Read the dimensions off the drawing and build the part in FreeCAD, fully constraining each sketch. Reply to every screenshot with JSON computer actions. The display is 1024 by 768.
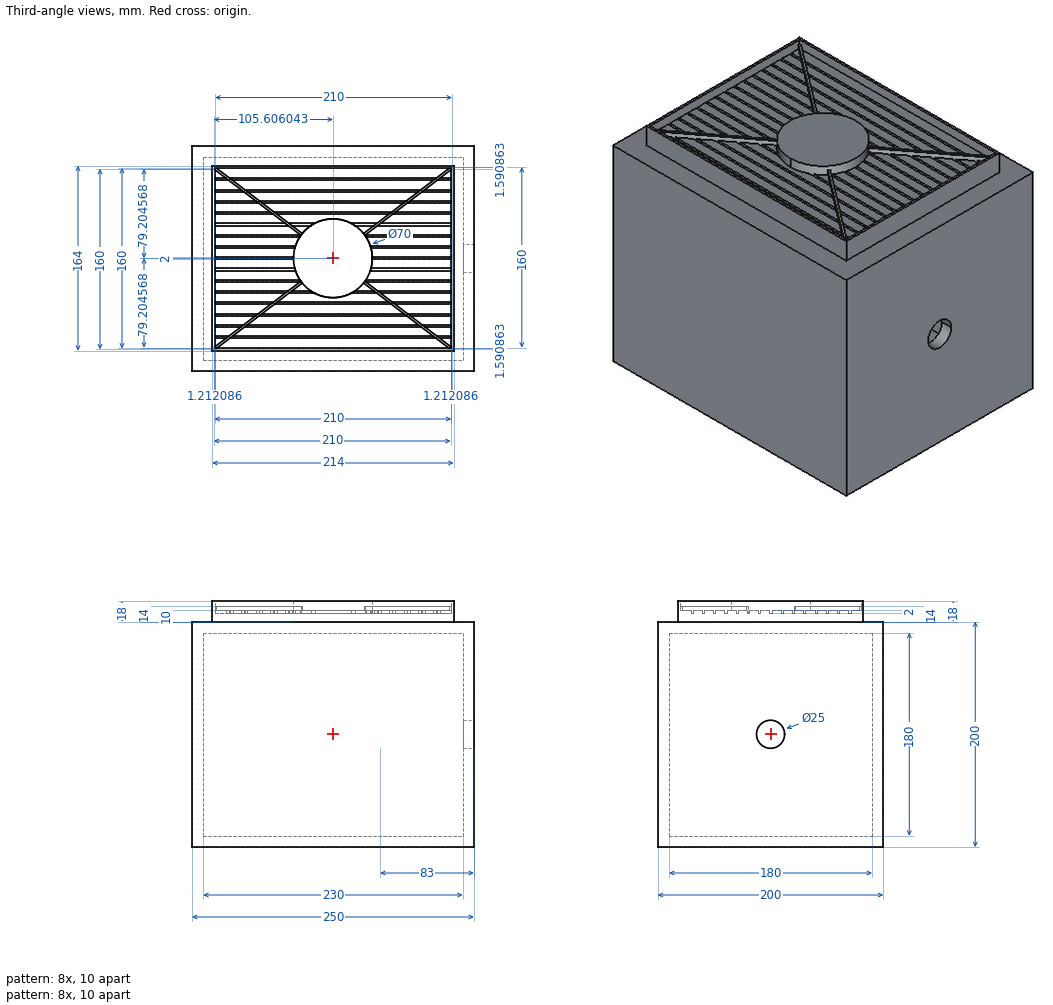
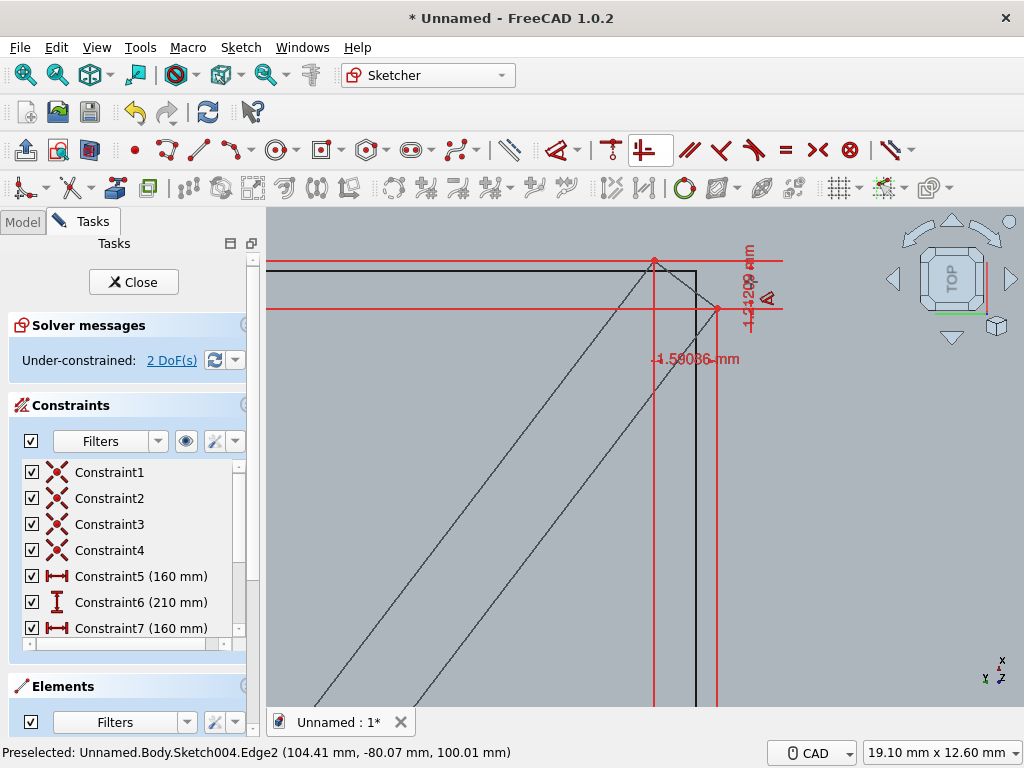
{"action": "scroll", "coordinate": [706, 288], "scroll_direction": "down", "scroll_amount": 16}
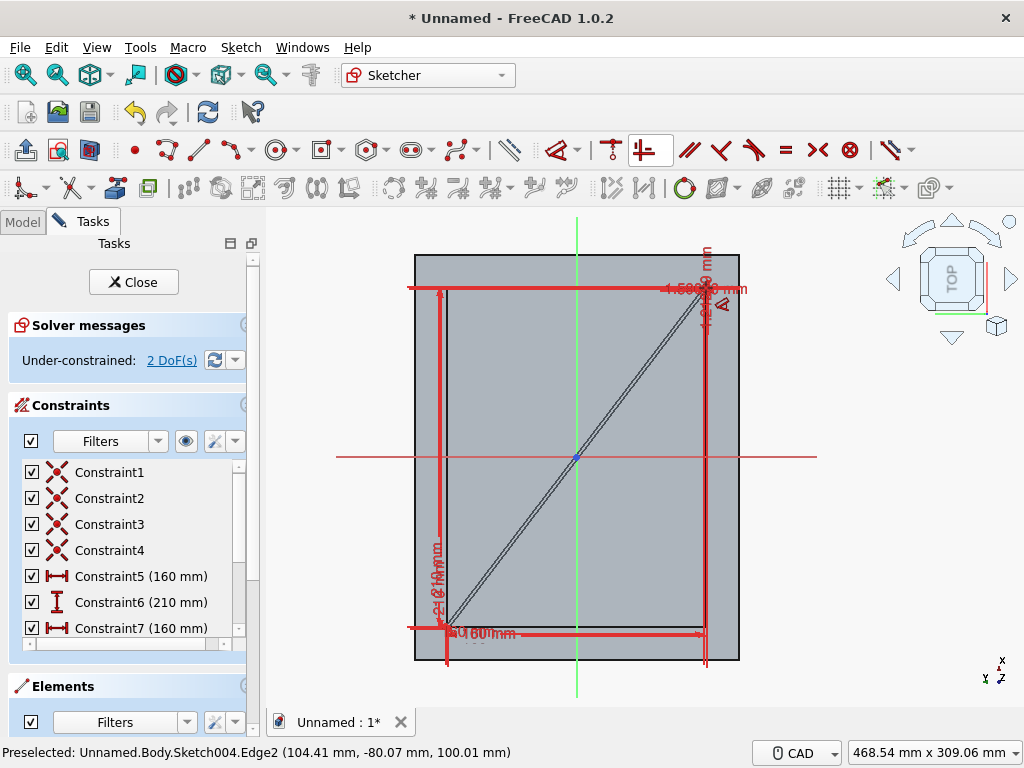
{"action": "scroll", "coordinate": [448, 629], "scroll_direction": "up", "scroll_amount": 7}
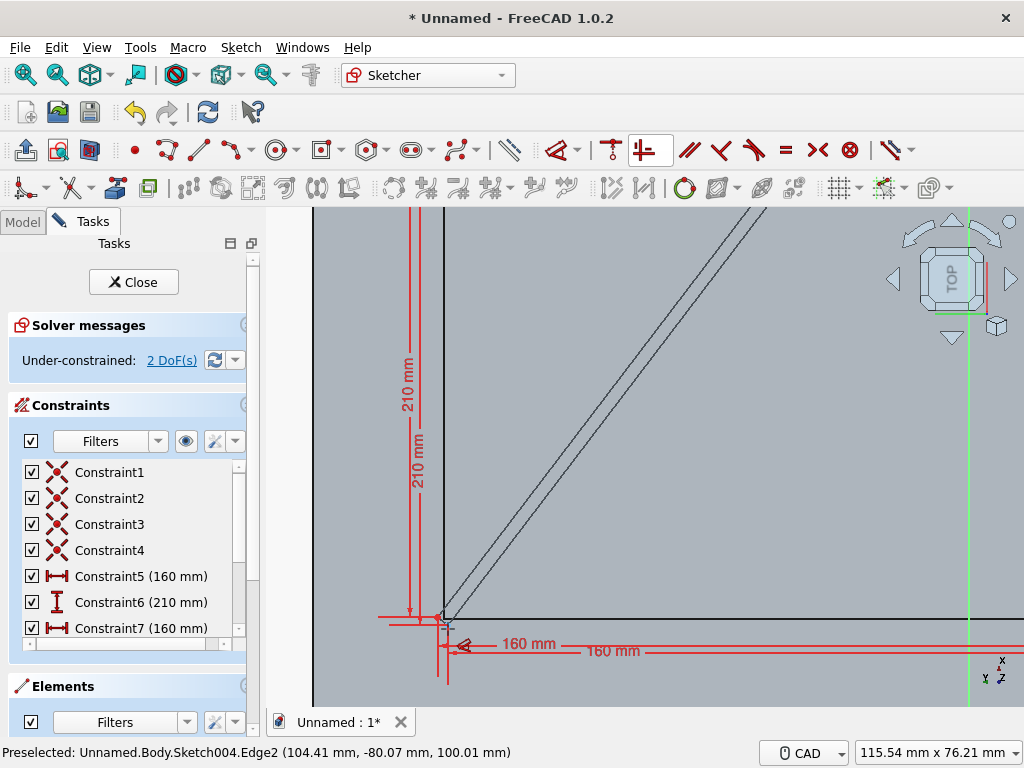
{"action": "left_click", "coordinate": [448, 625]}
{"action": "left_click", "coordinate": [748, 659]}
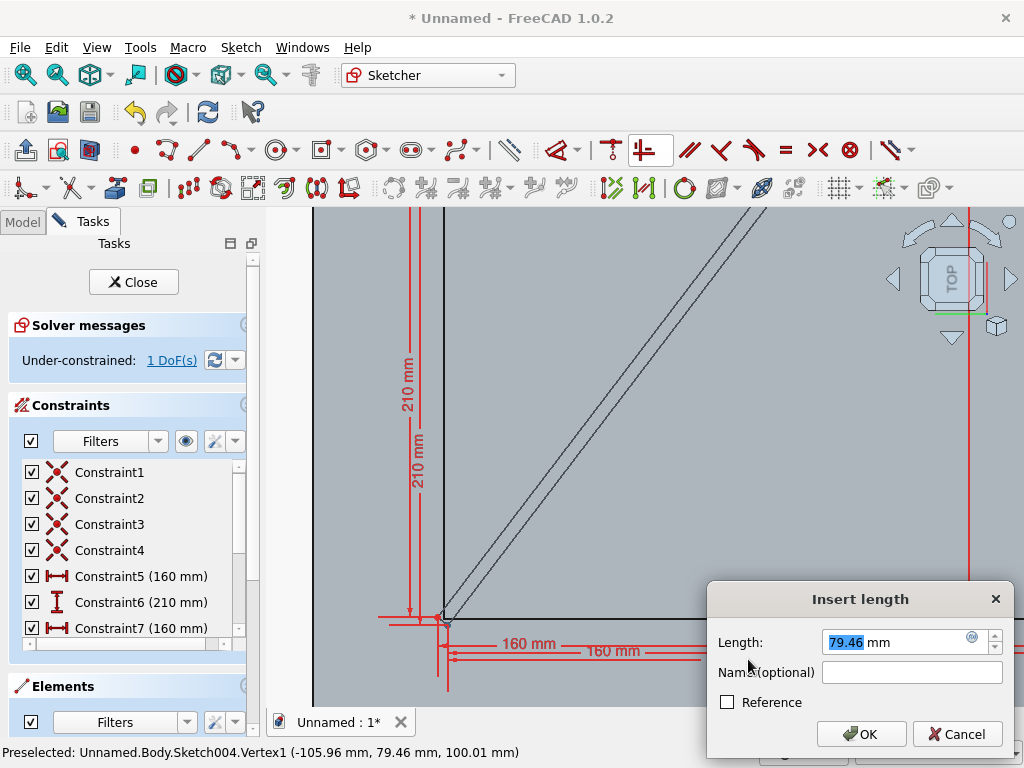
{"action": "type", "text": "79.204568"}
{"action": "key", "text": "Return"}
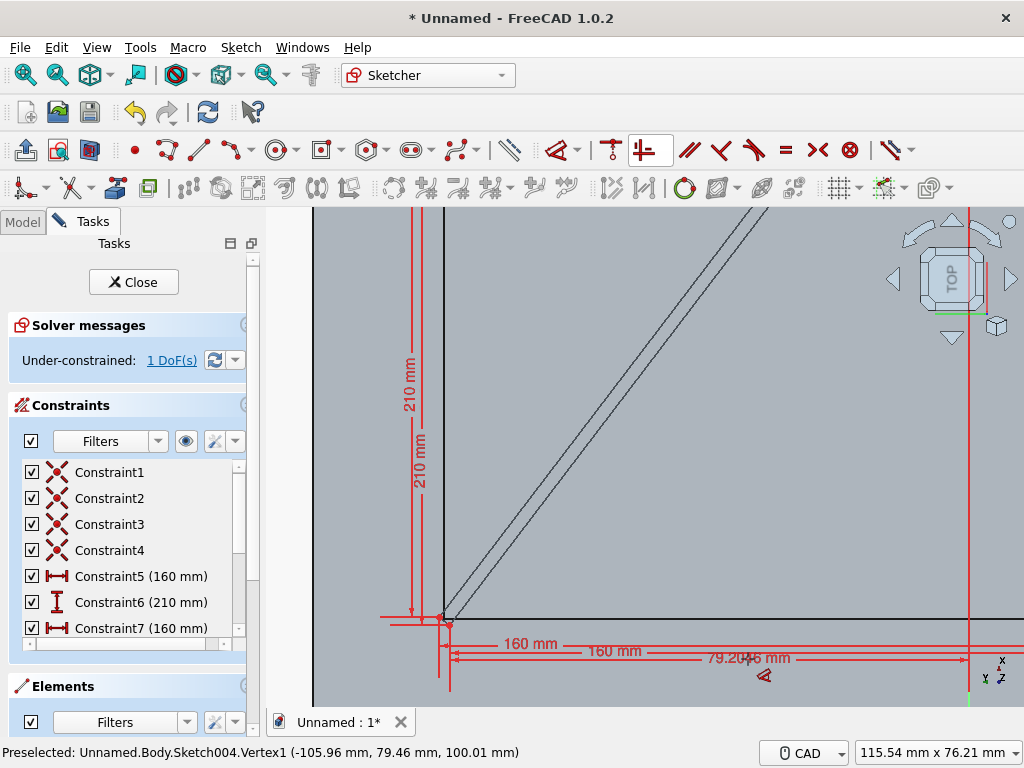
{"action": "left_click", "coordinate": [450, 625]}
{"action": "left_click", "coordinate": [416, 430]}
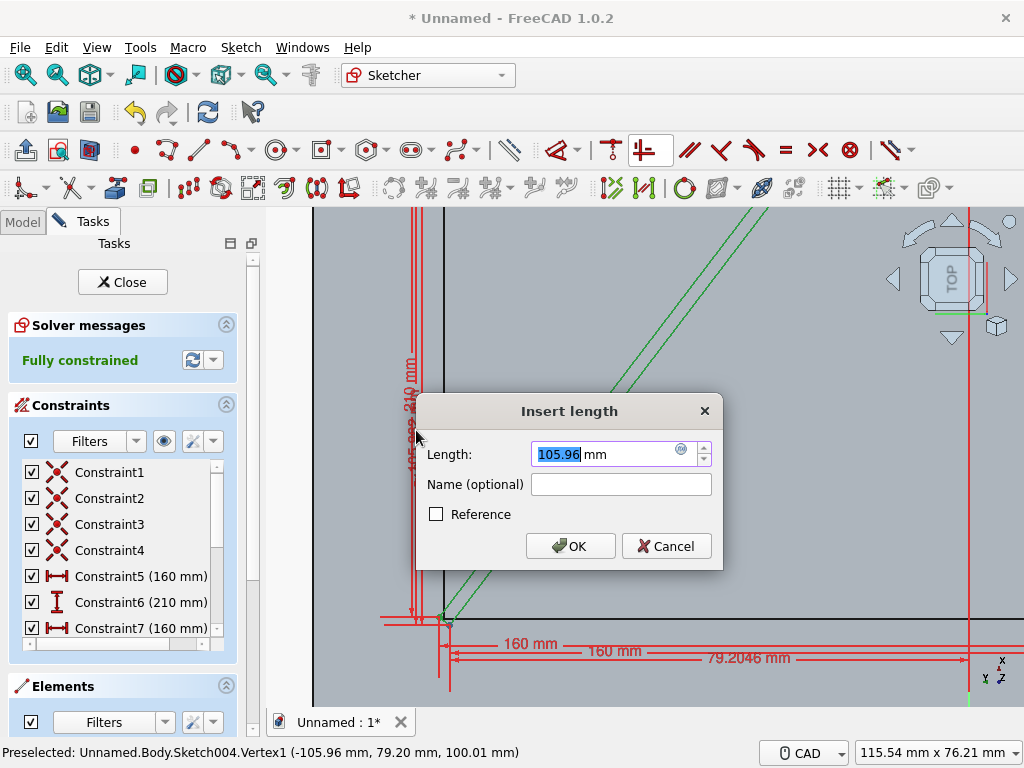
{"action": "type", "text": "105.606043"}
{"action": "key", "text": "Return"}
{"action": "key", "text": "Escape"}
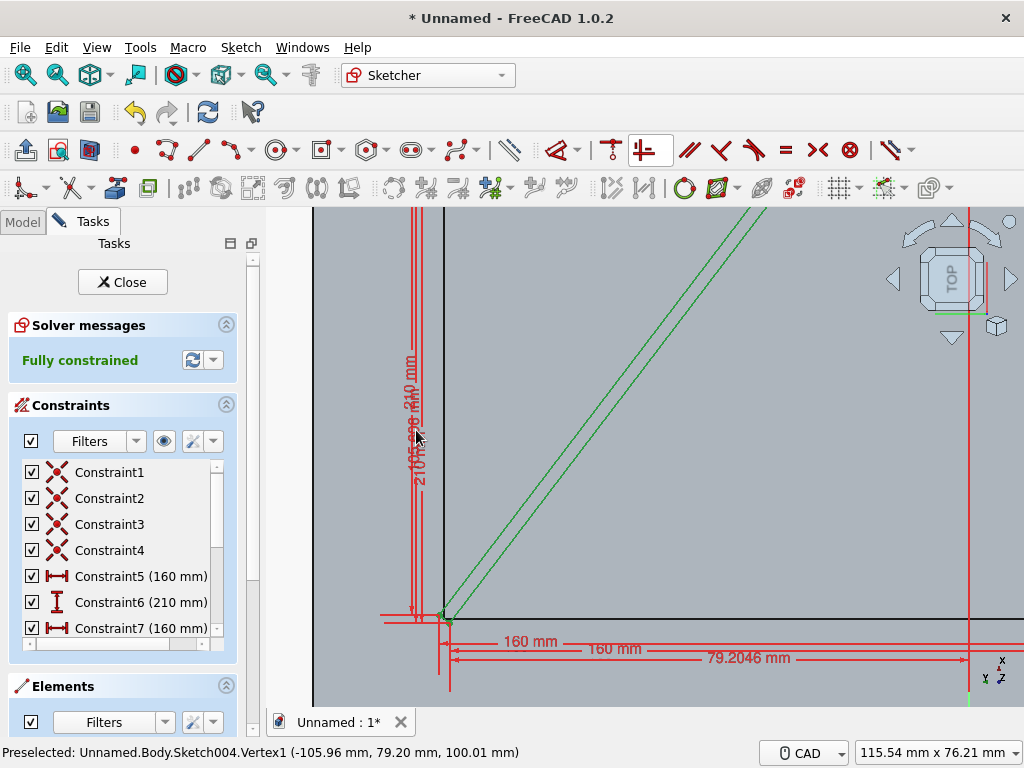
{"action": "left_click", "coordinate": [123, 282]}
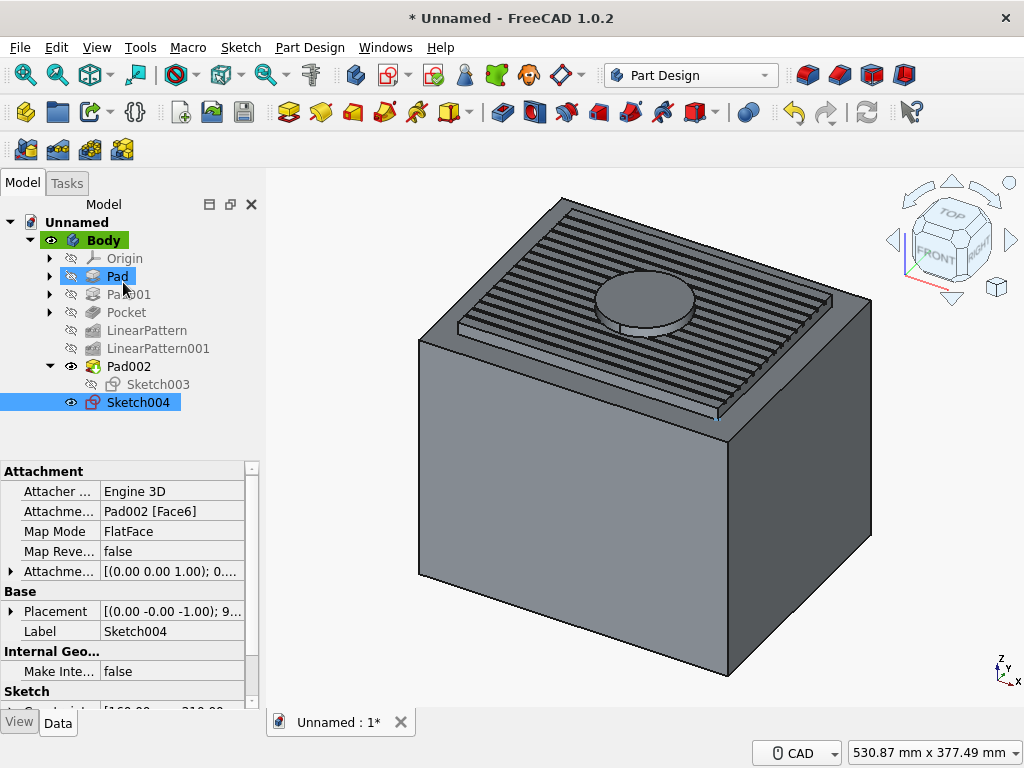
{"action": "left_click", "coordinate": [290, 112]}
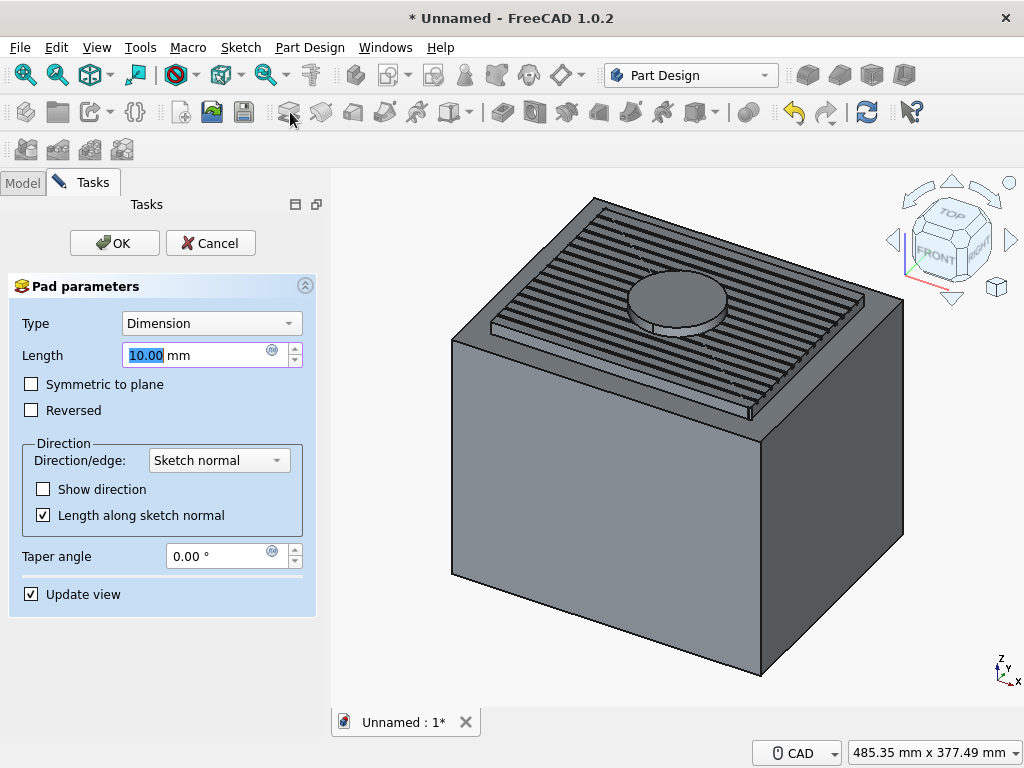
{"action": "type", "text": "14"}
{"action": "key", "text": "Tab"}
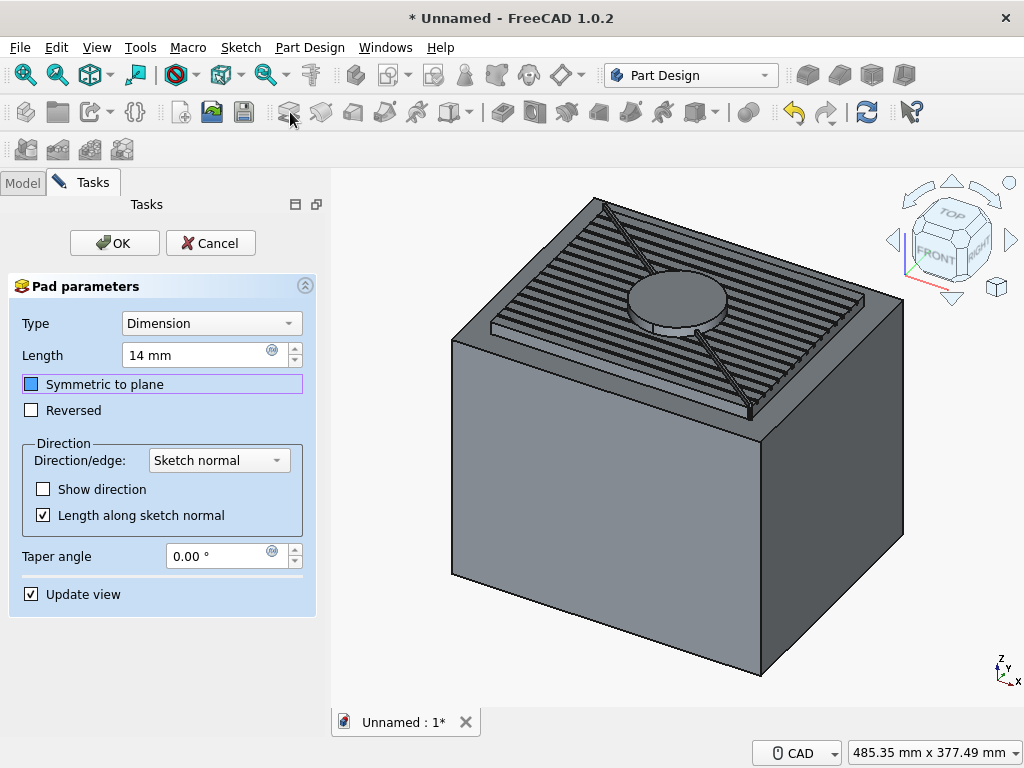
{"action": "left_click", "coordinate": [115, 243]}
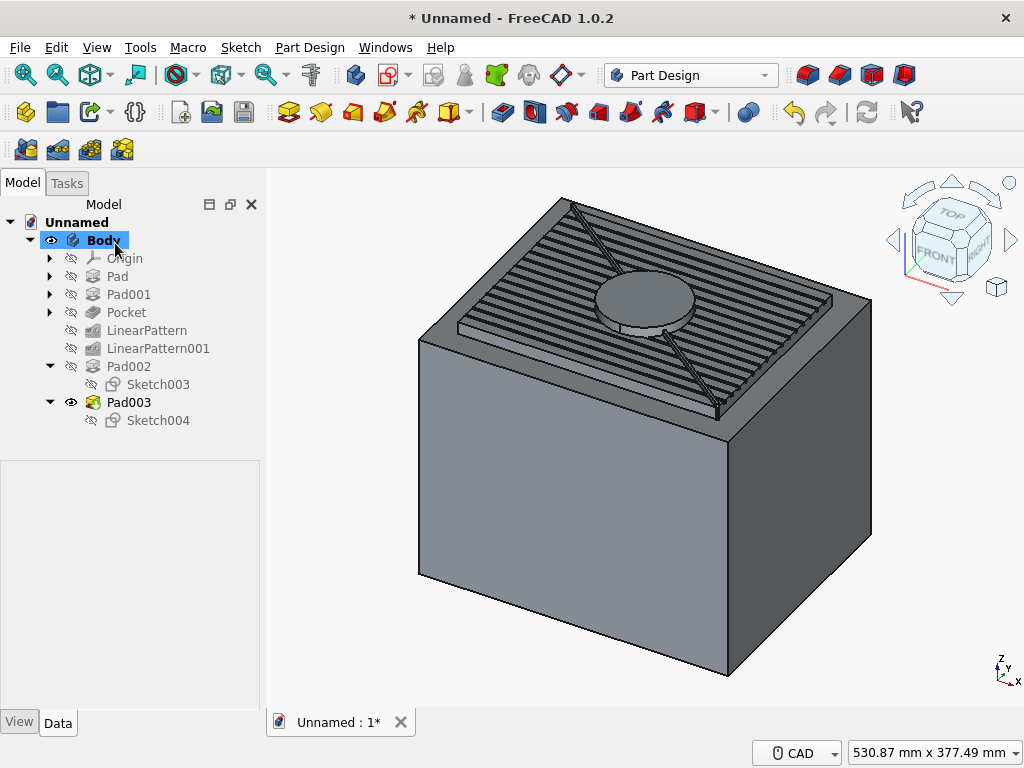
{"action": "left_click", "coordinate": [451, 336]}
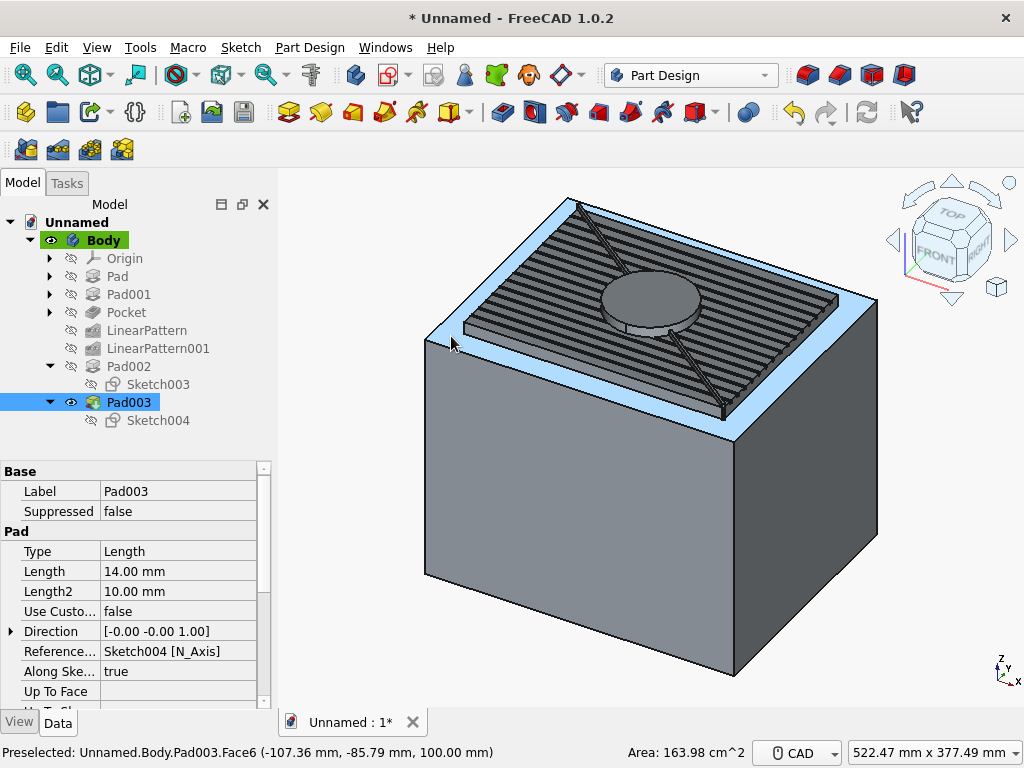
{"action": "left_click", "coordinate": [388, 76]}